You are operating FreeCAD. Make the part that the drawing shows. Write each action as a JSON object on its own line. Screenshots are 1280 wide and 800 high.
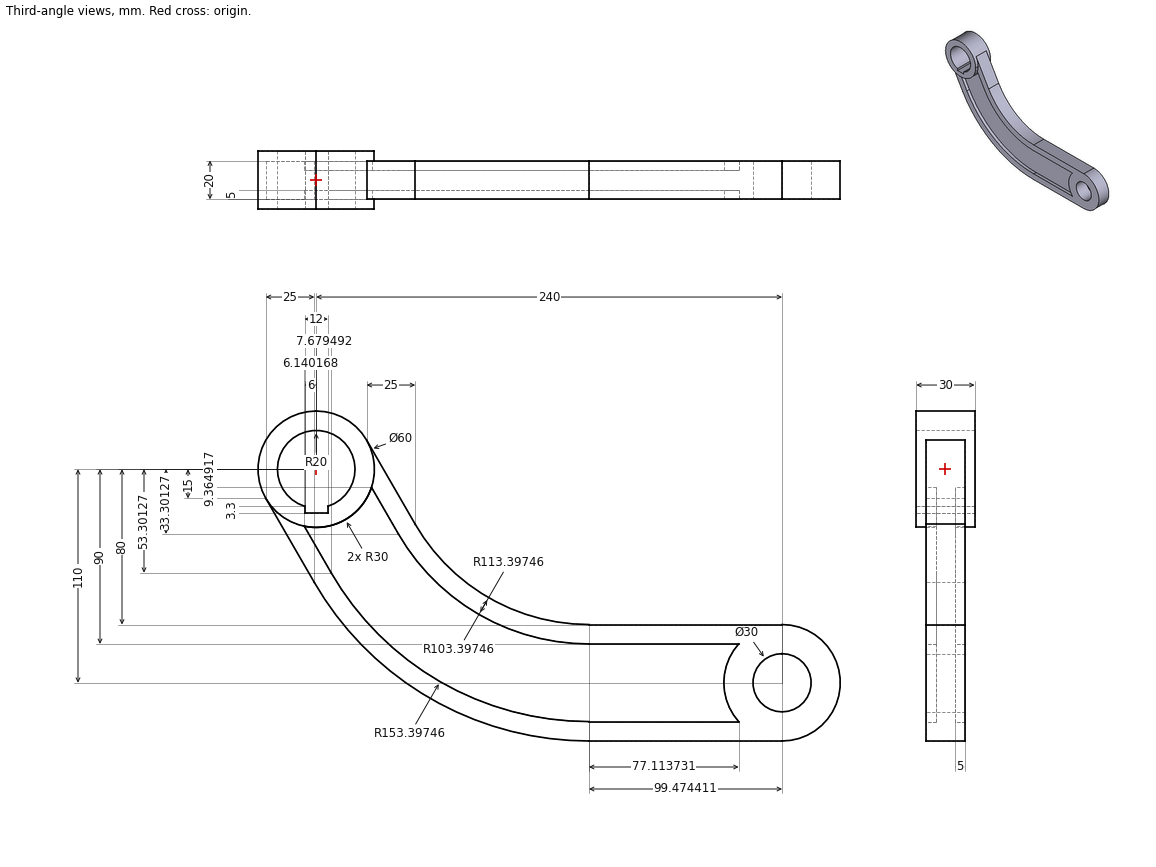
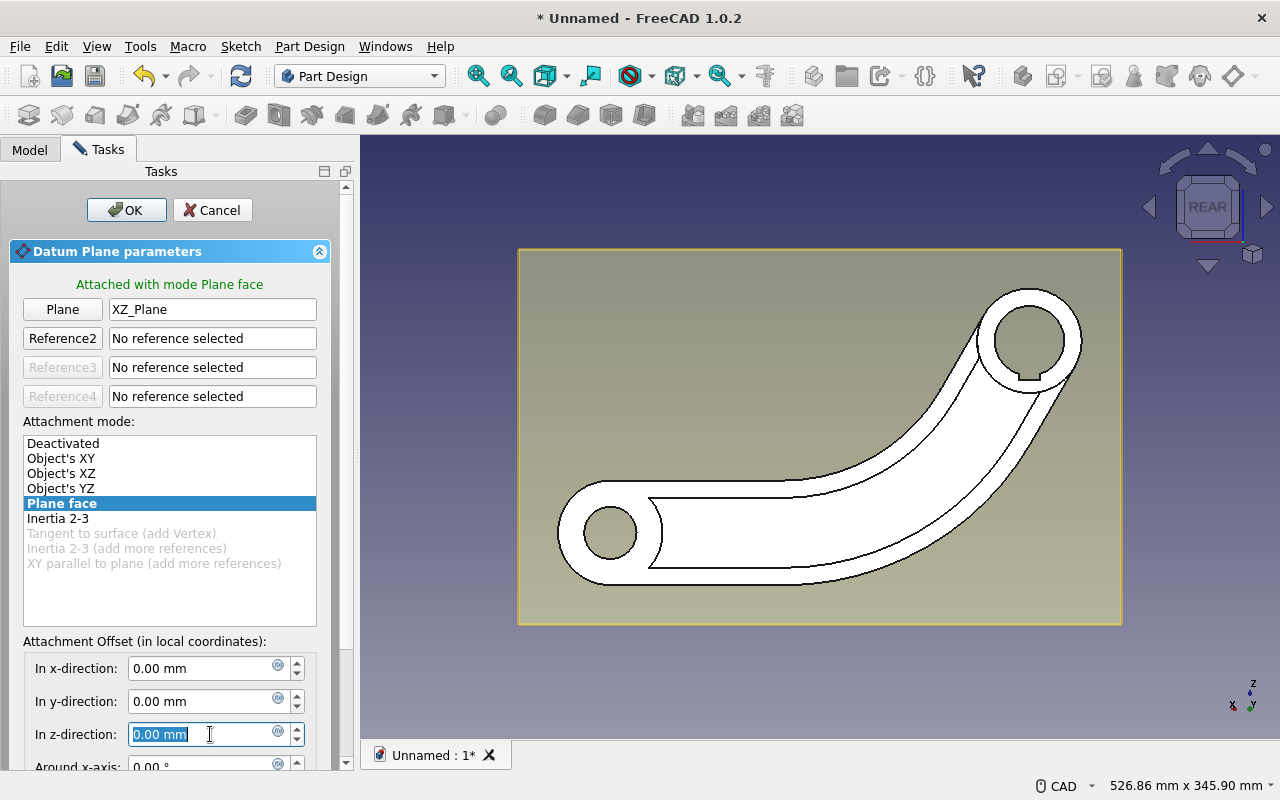
{"action": "type", "text": "5"}
{"action": "key", "text": "Tab"}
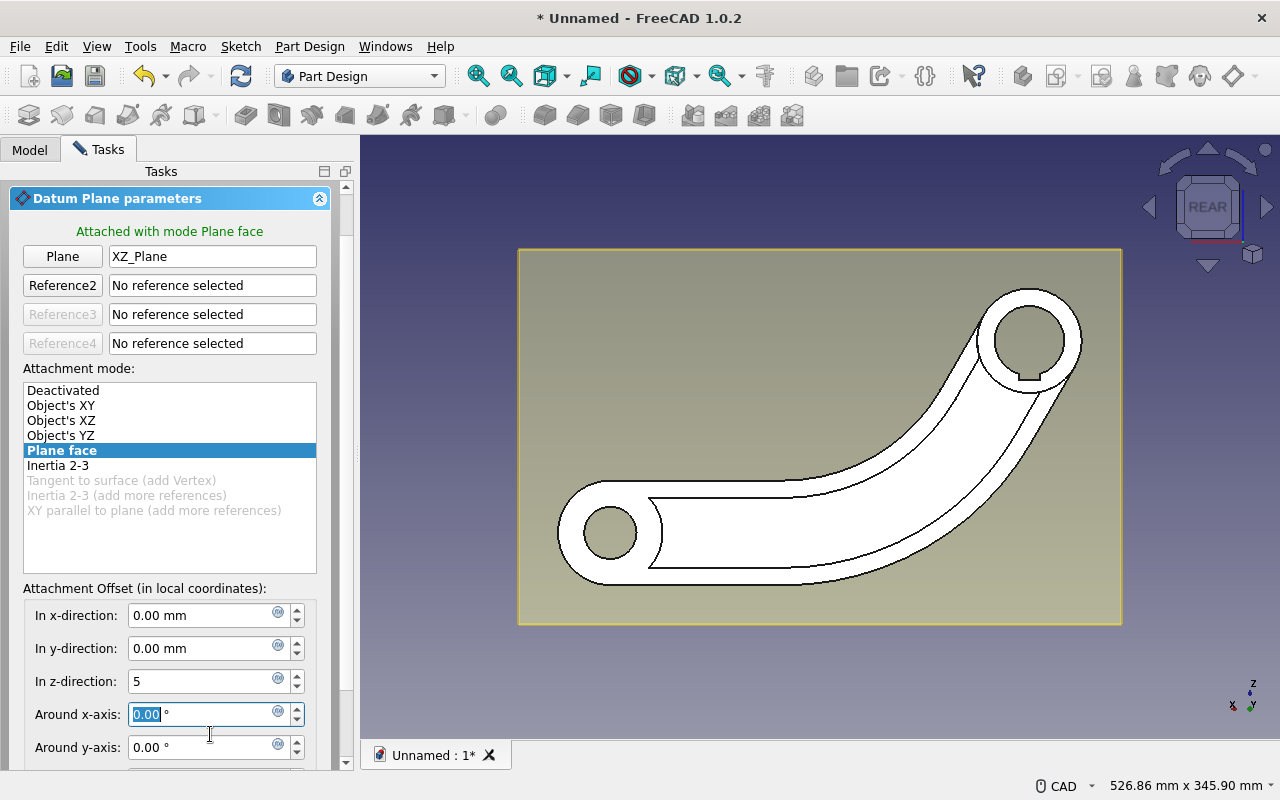
{"action": "scroll", "coordinate": [346, 476], "scroll_direction": "up", "scroll_amount": 2}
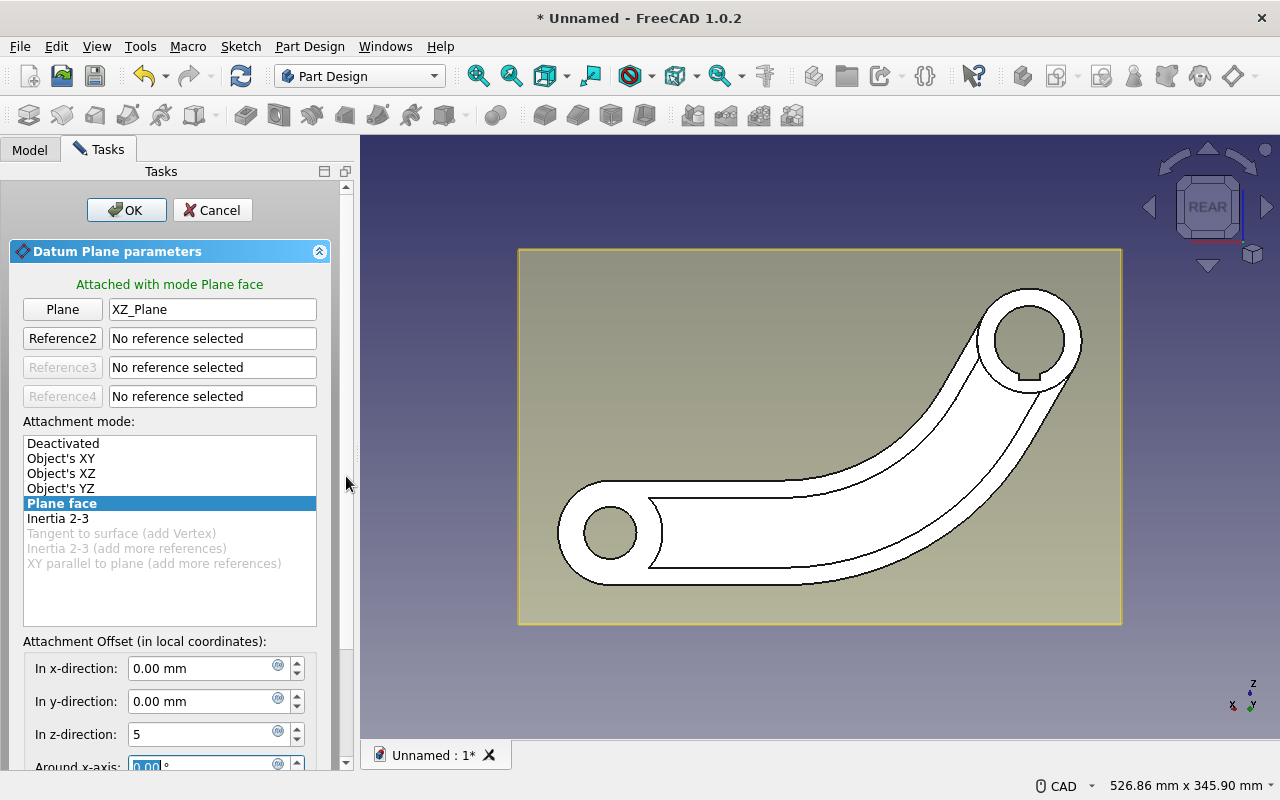
{"action": "left_click", "coordinate": [127, 210]}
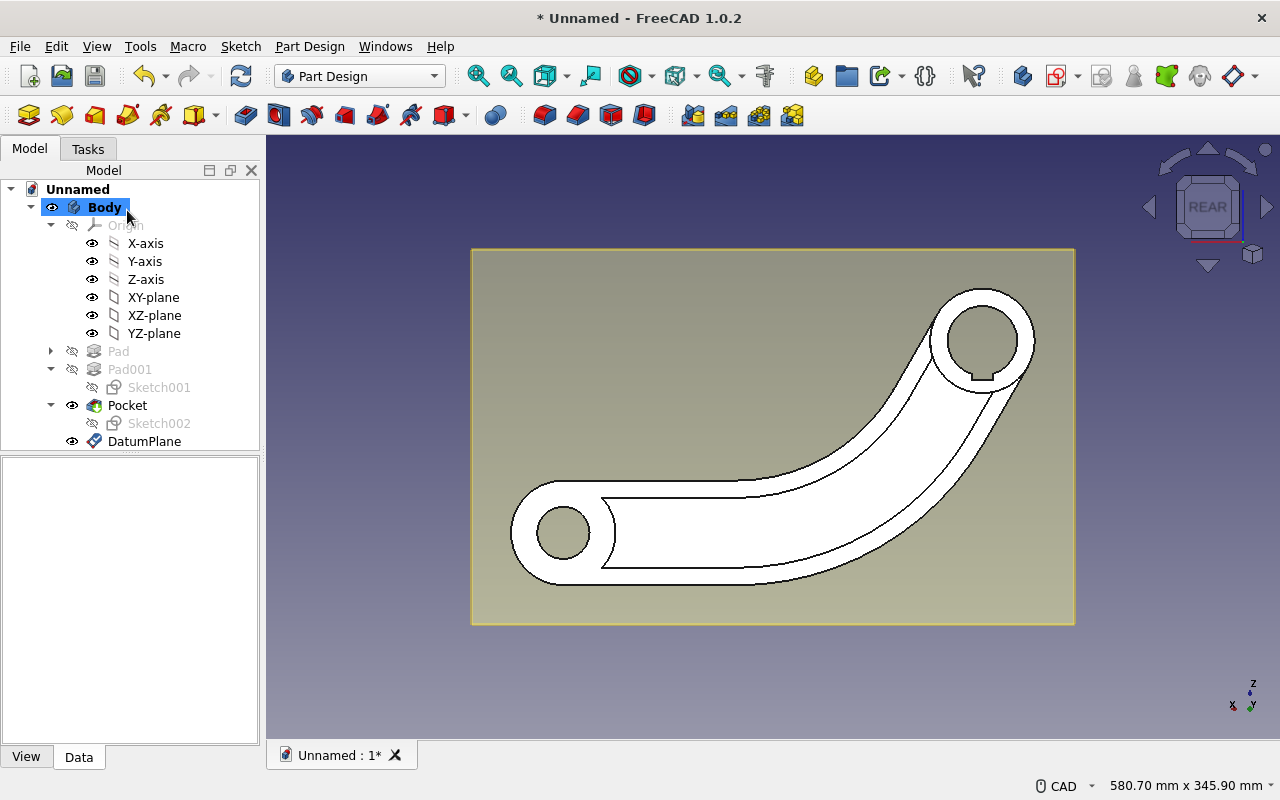
{"action": "left_click", "coordinate": [117, 441]}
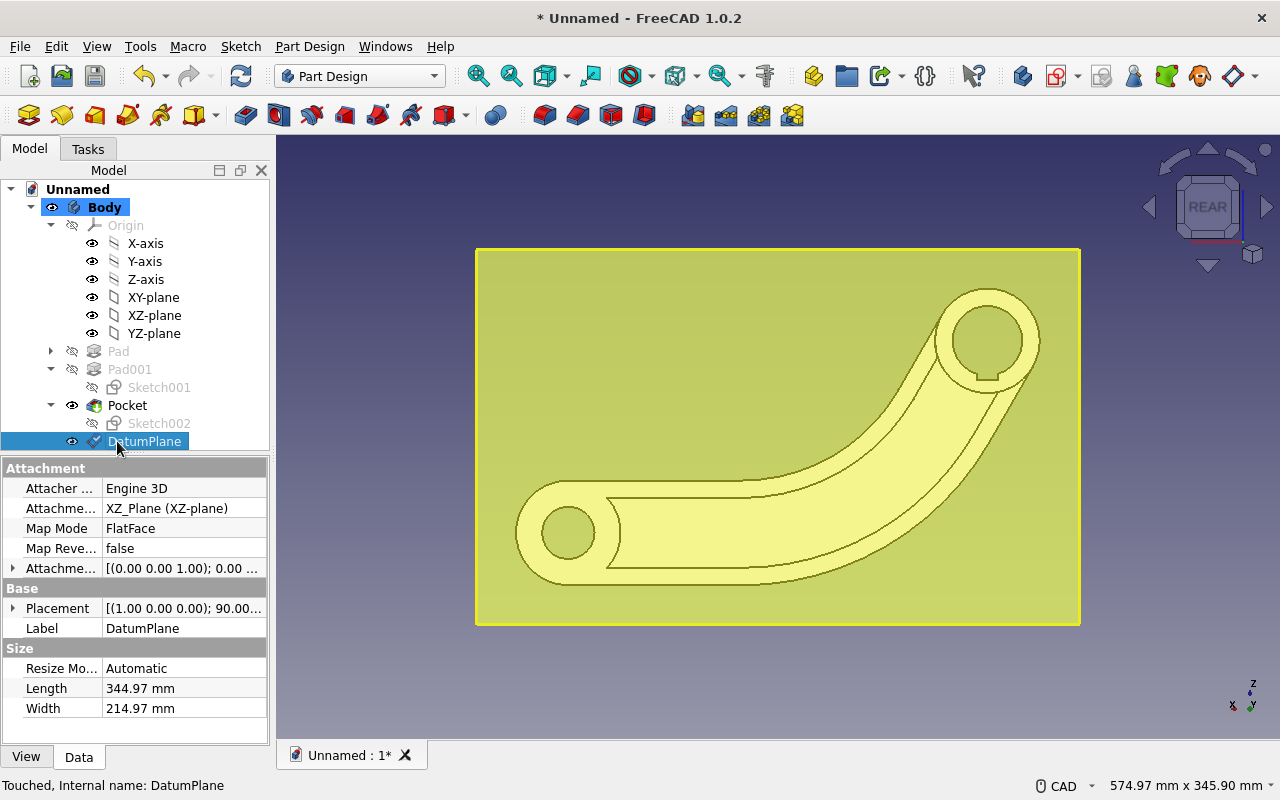
{"action": "left_click", "coordinate": [1056, 76]}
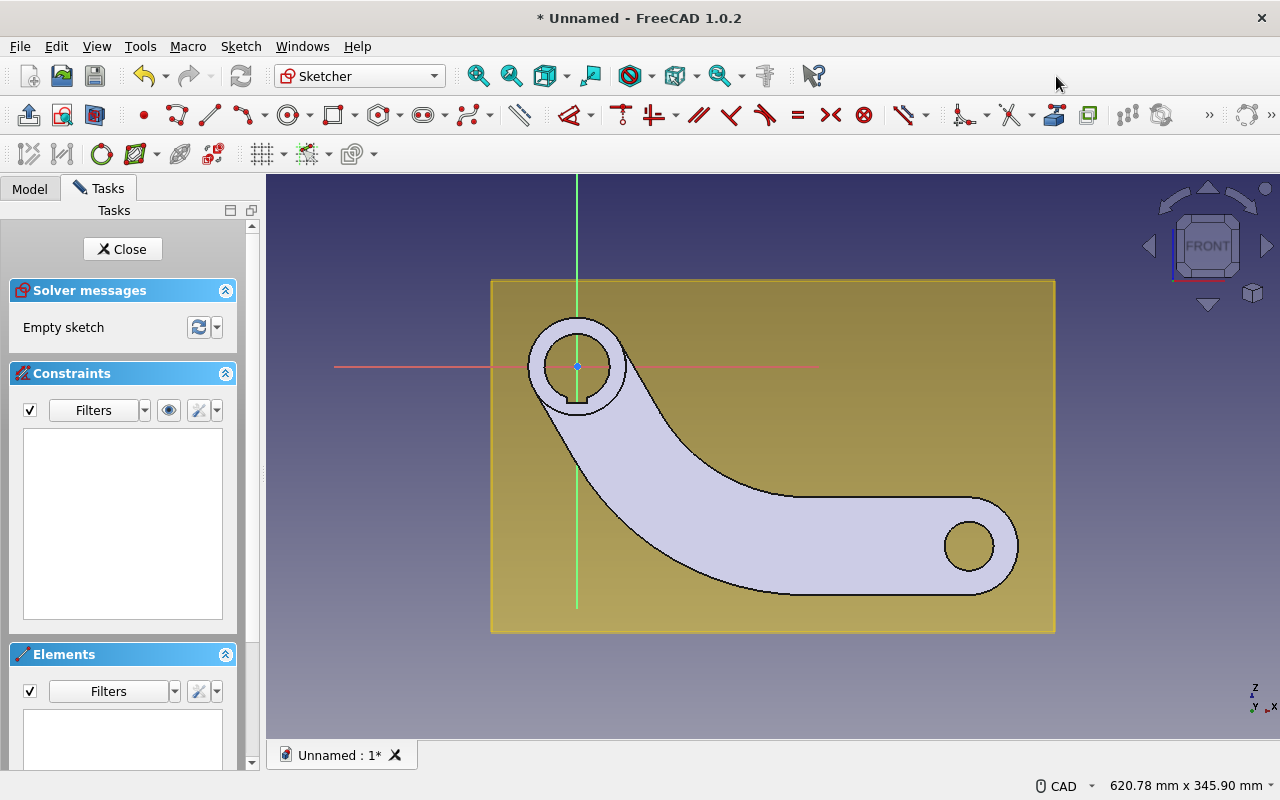
{"action": "left_click", "coordinate": [95, 116]}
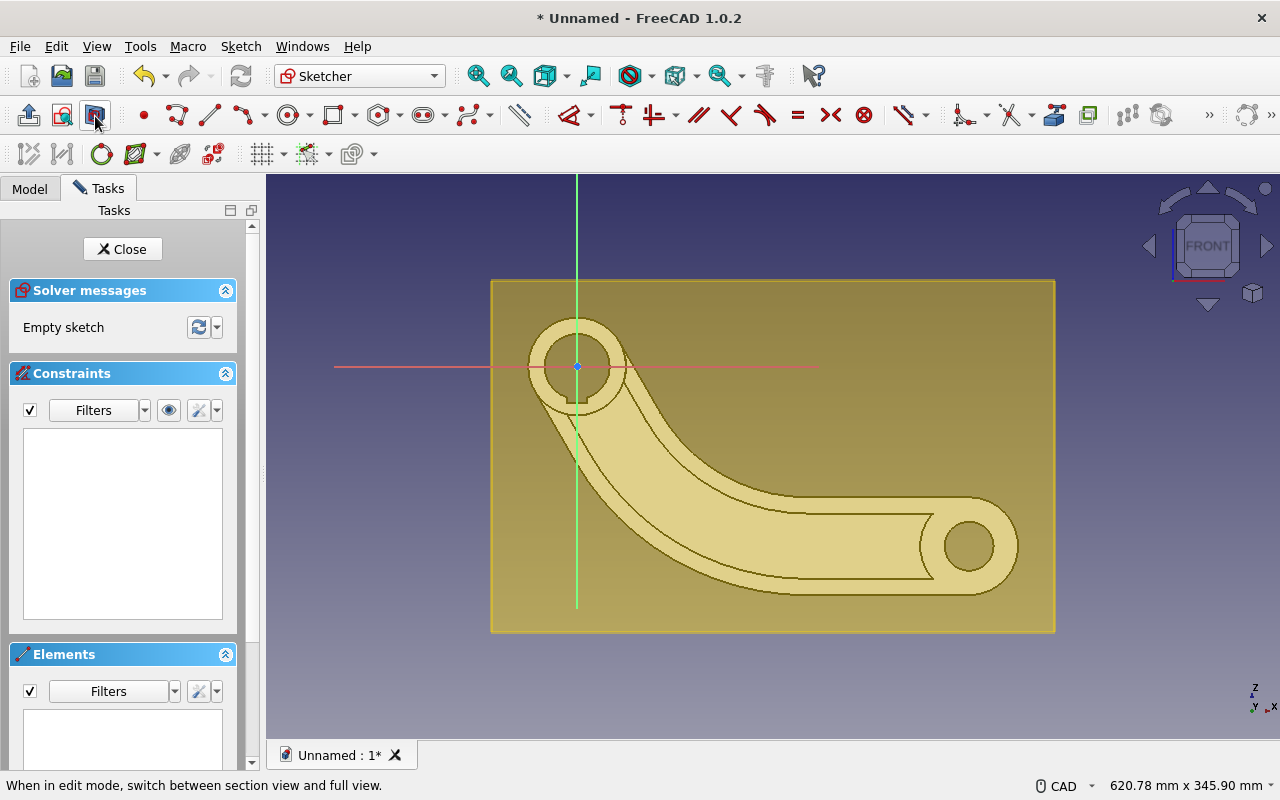
{"action": "scroll", "coordinate": [842, 506], "scroll_direction": "up", "scroll_amount": 2}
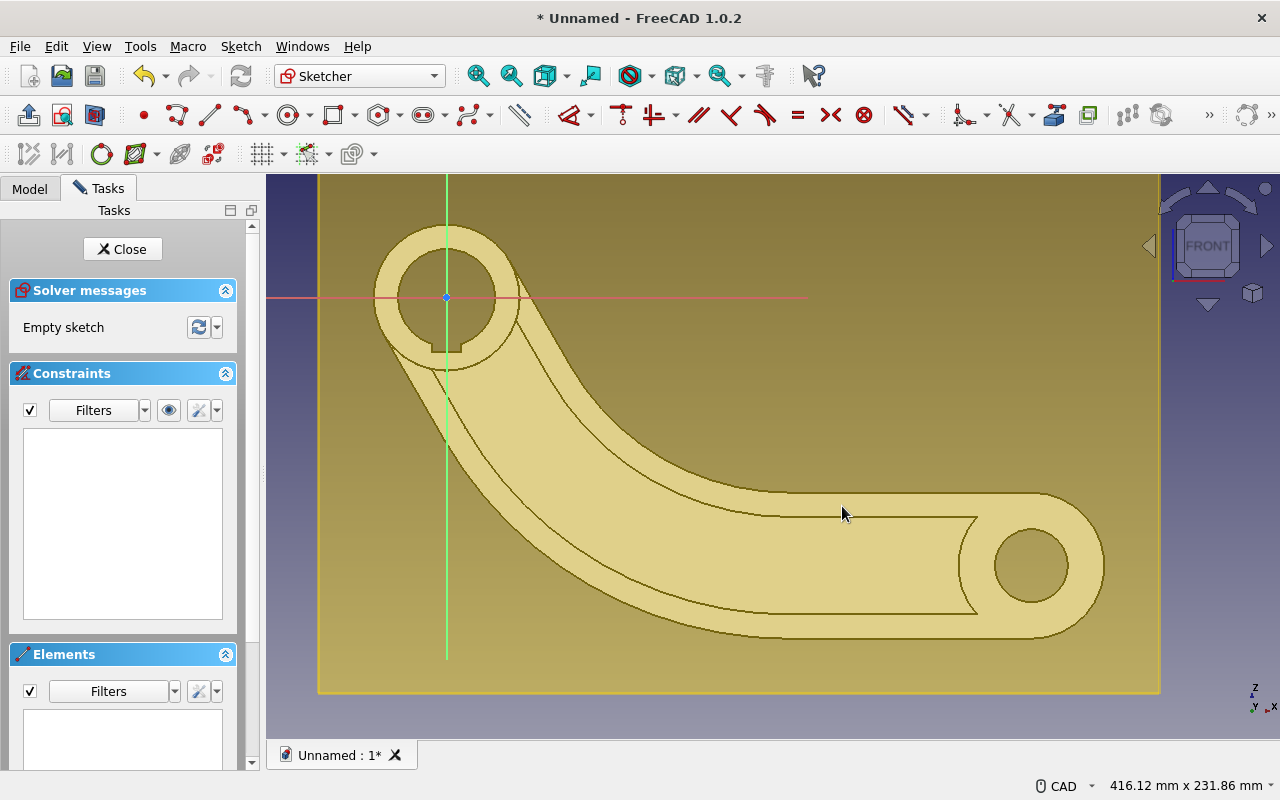
{"action": "left_click", "coordinate": [210, 116]}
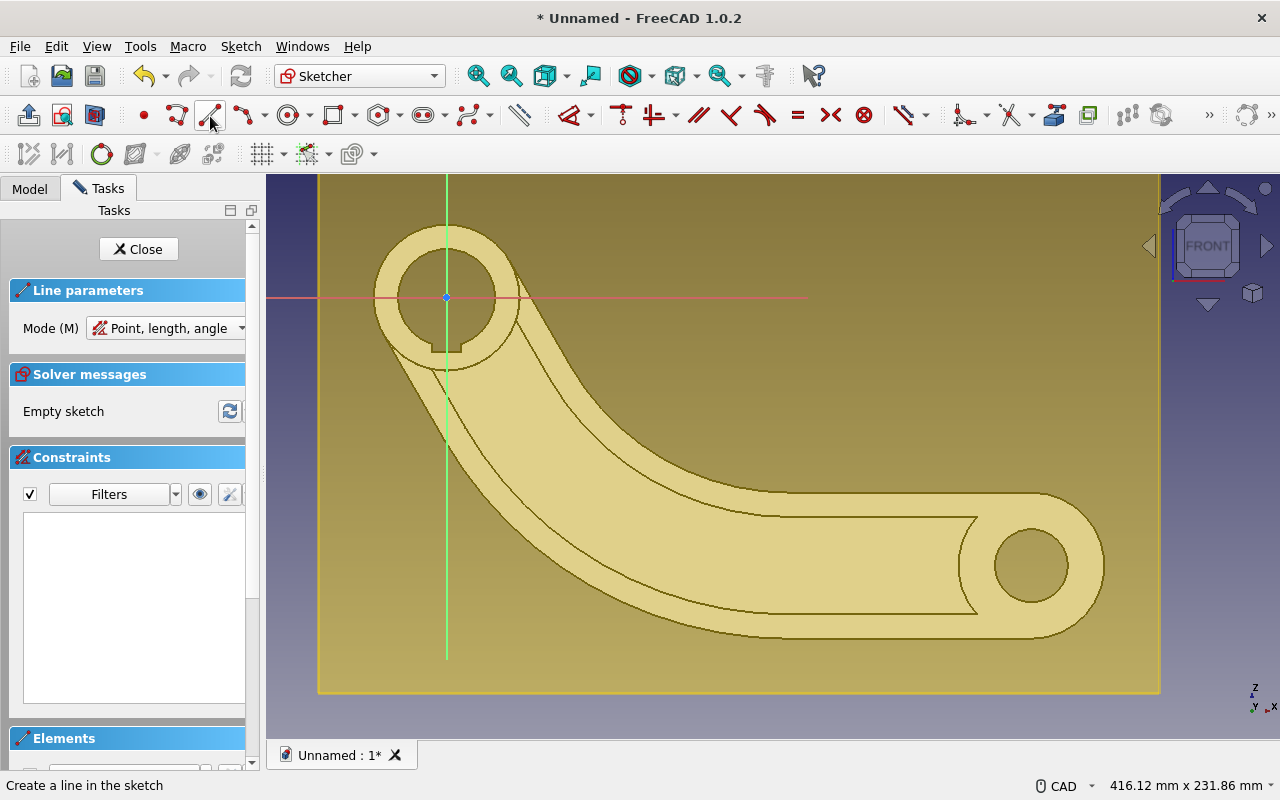
{"action": "left_click", "coordinate": [977, 517]}
{"action": "left_click", "coordinate": [789, 517]}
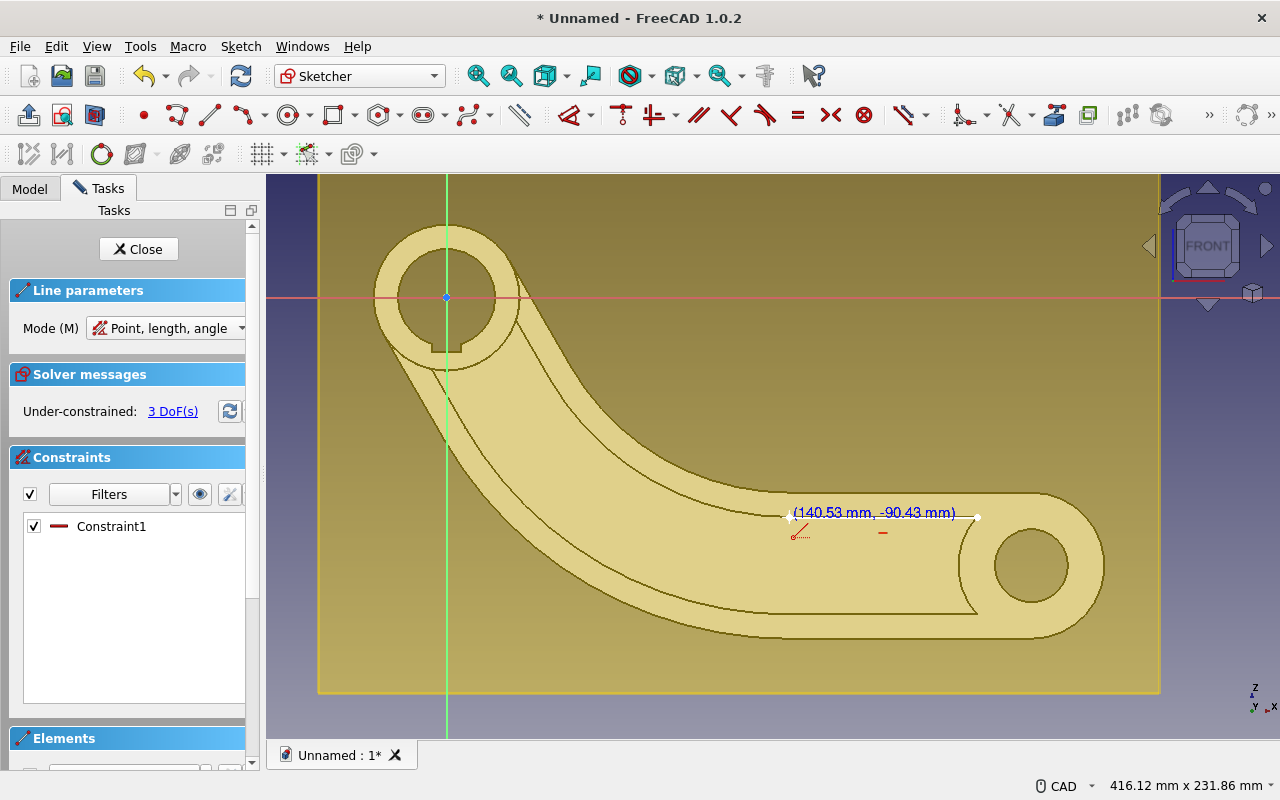
{"action": "left_click", "coordinate": [550, 379]}
{"action": "left_click", "coordinate": [516, 320]}